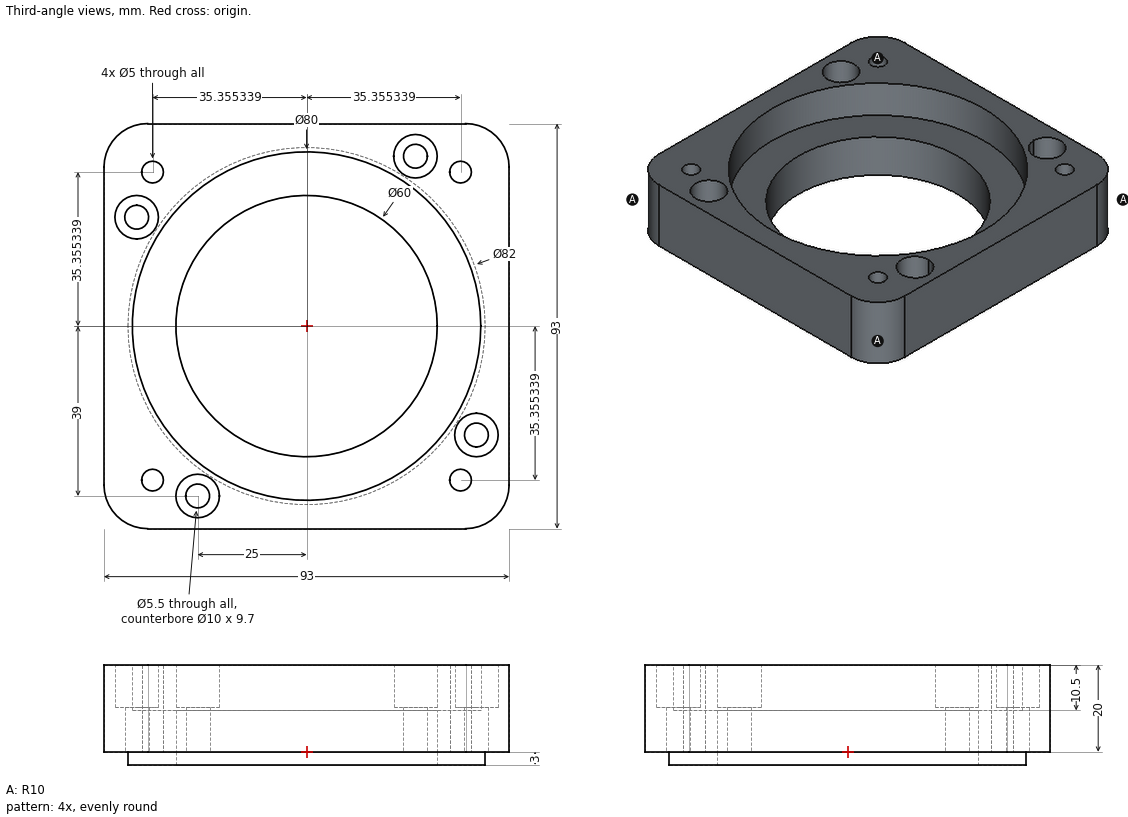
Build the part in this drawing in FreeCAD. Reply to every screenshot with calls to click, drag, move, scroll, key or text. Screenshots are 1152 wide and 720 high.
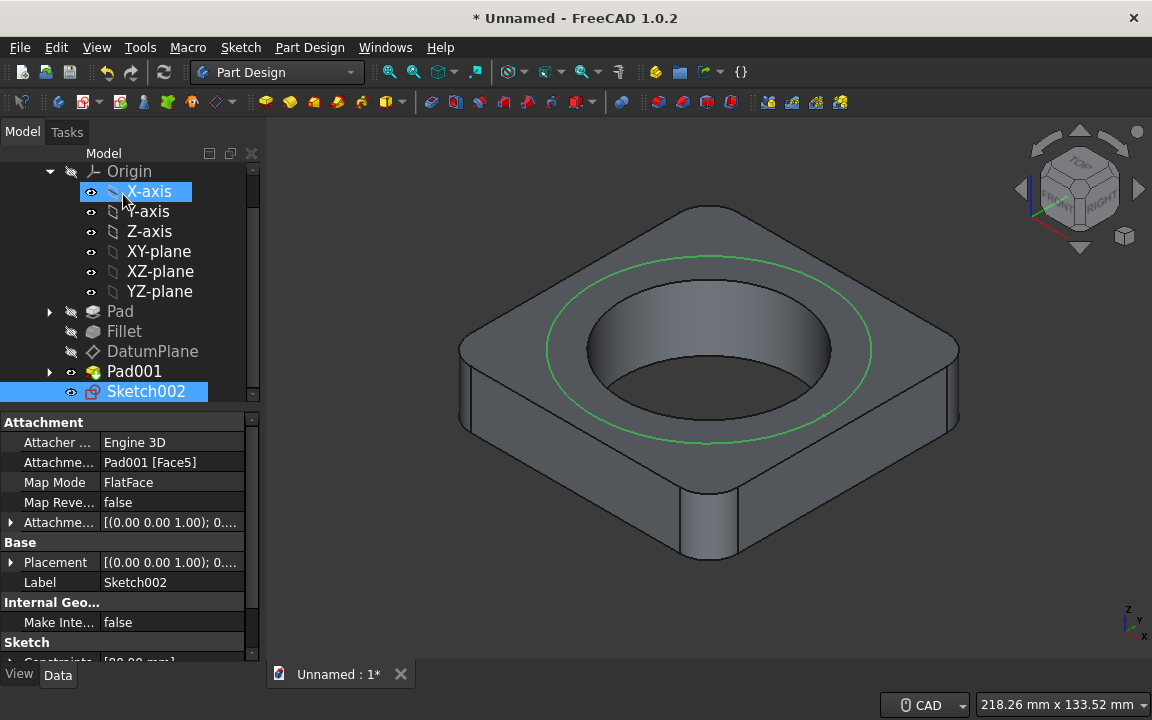
click(432, 102)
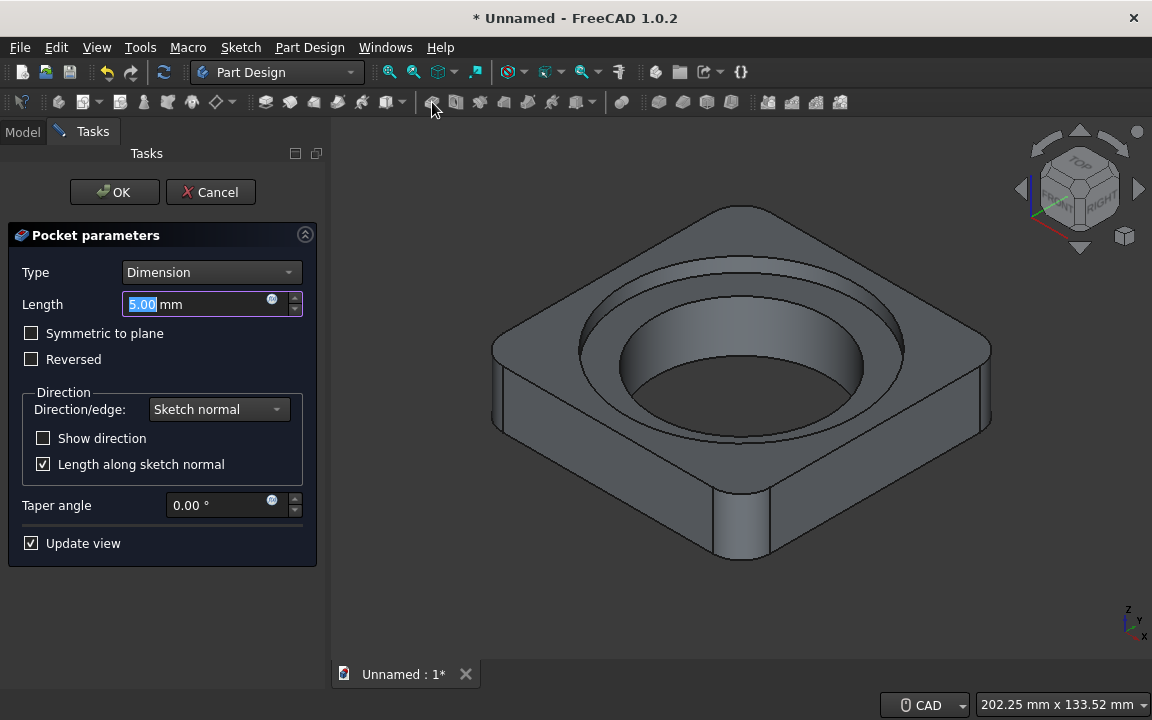
text(10.5)
key(Tab)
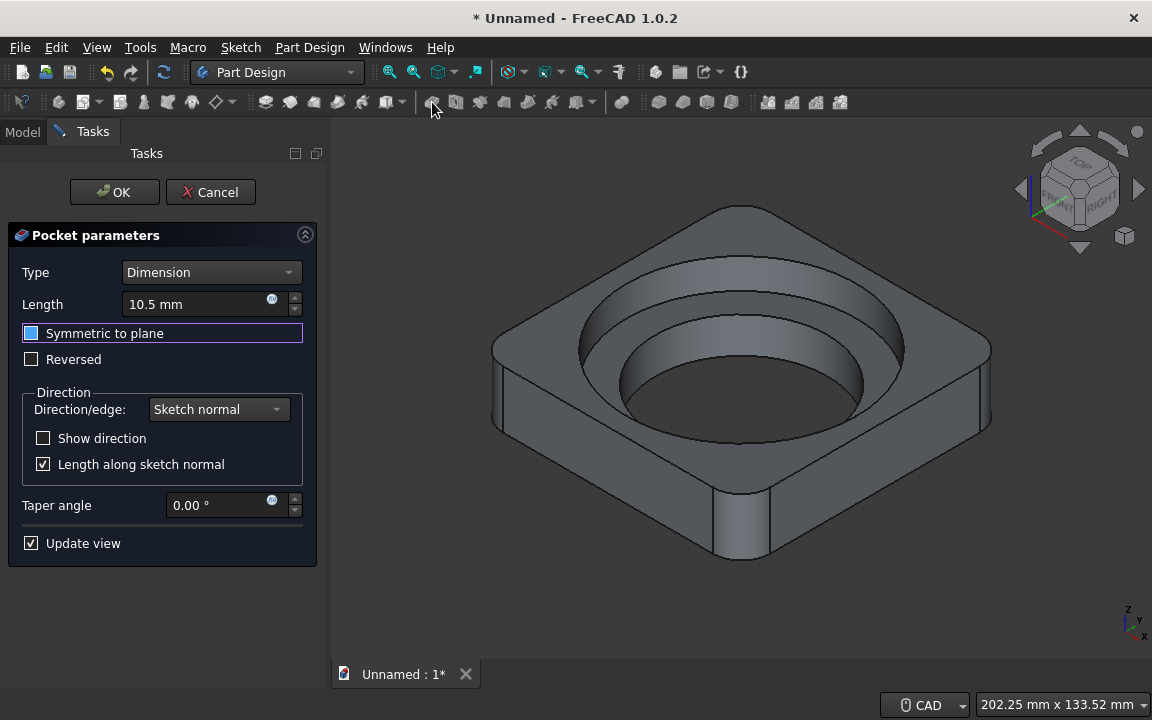
click(115, 192)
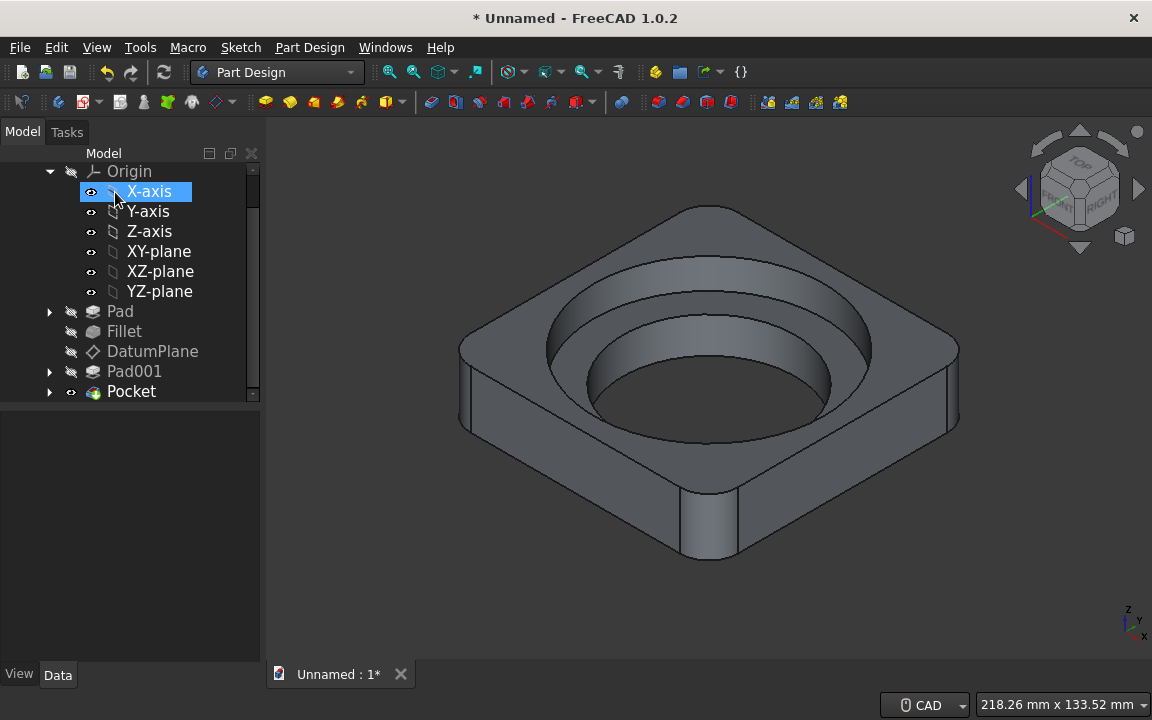
click(671, 459)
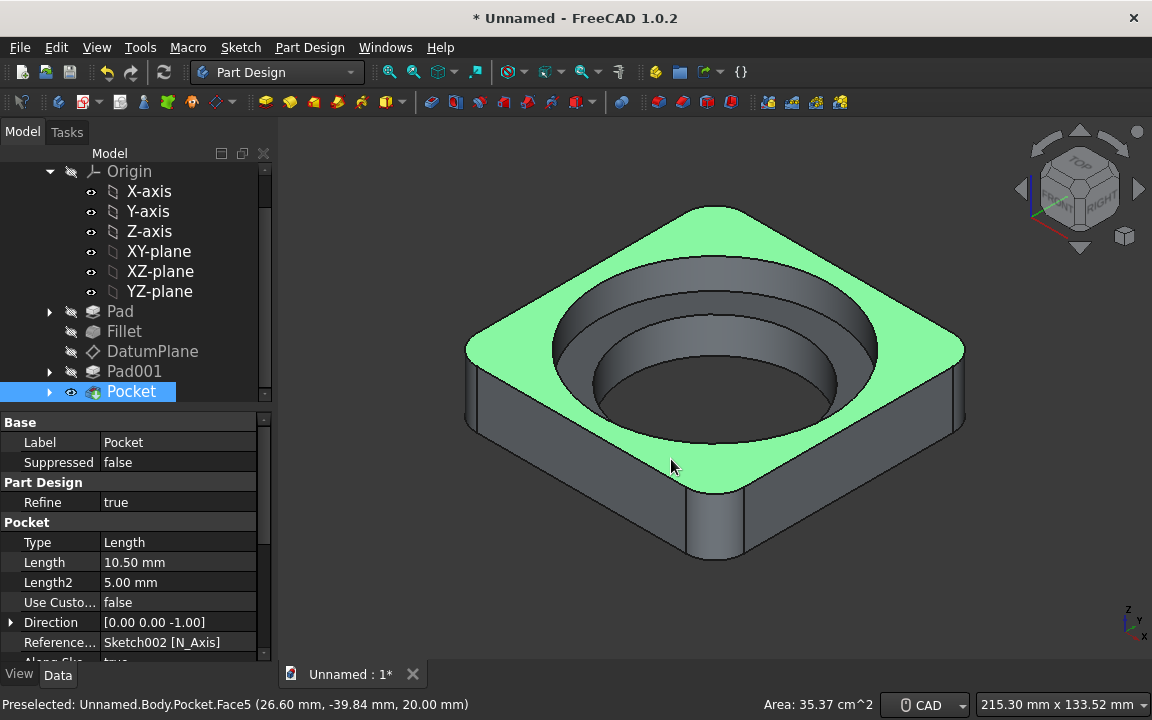
click(84, 102)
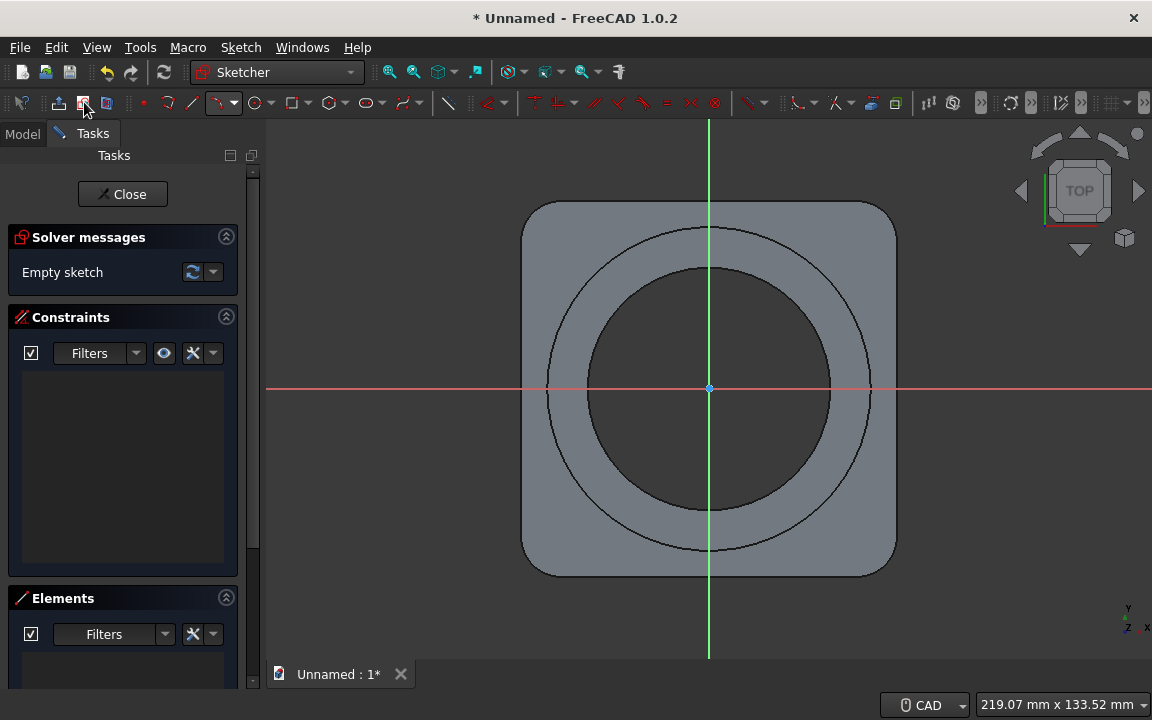
click(256, 104)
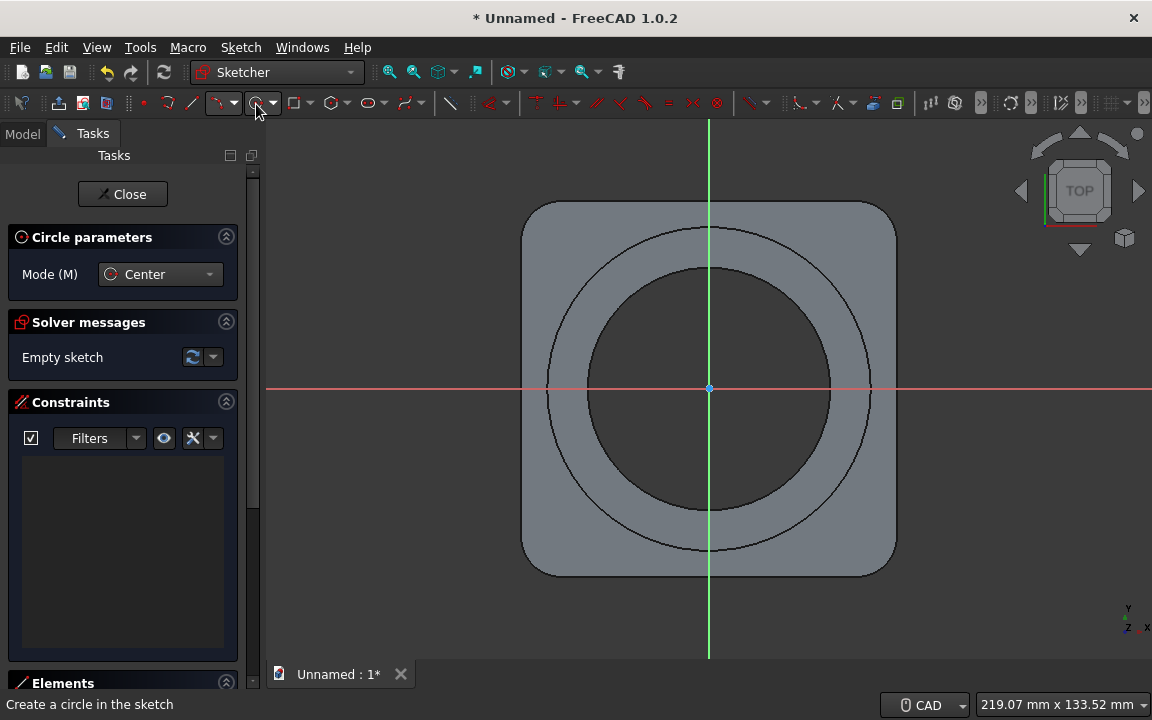
scroll(566, 246, up, 5)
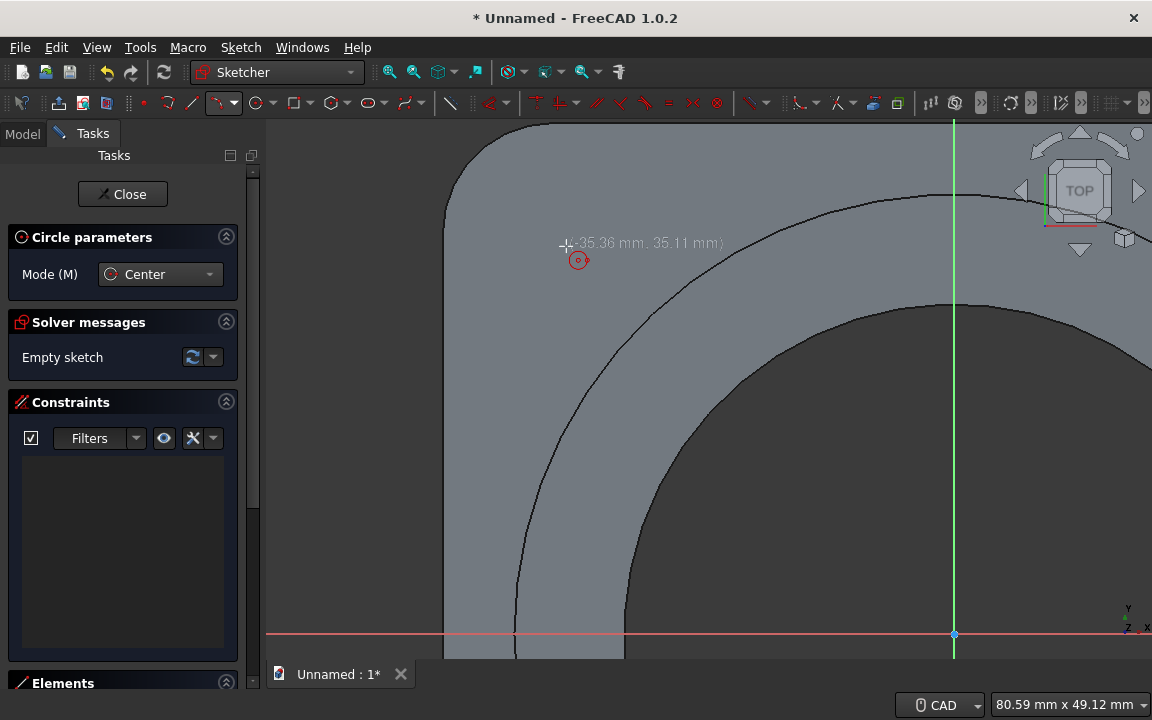
click(565, 246)
click(585, 226)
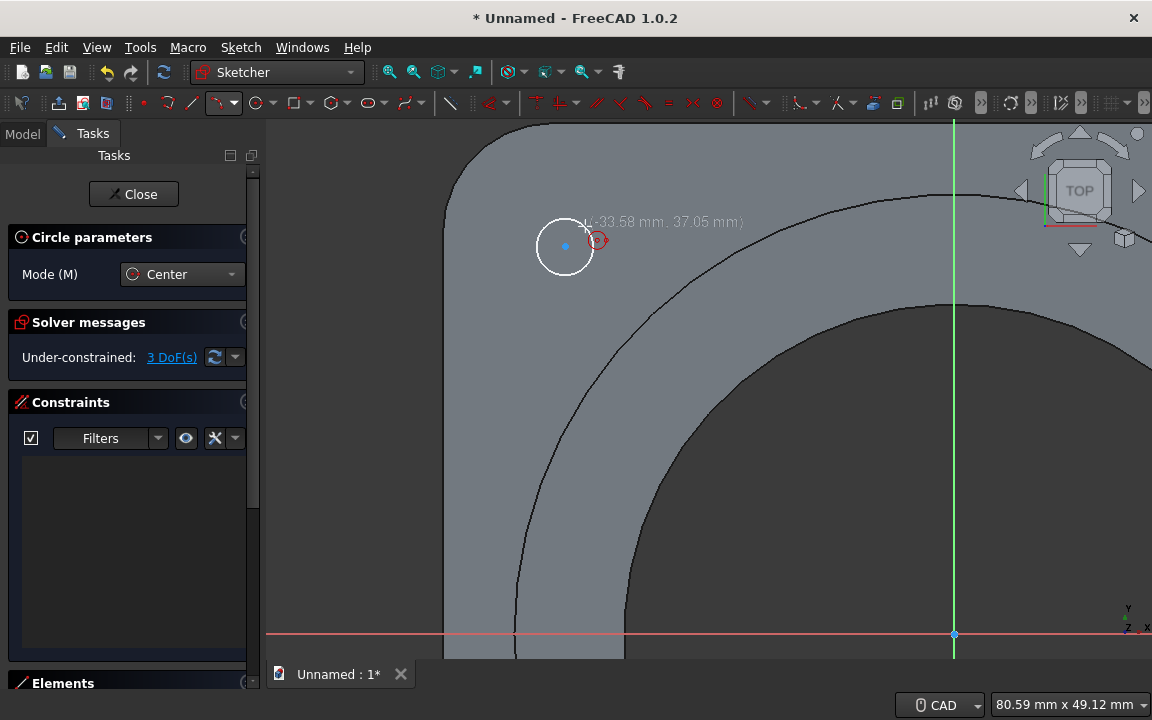
scroll(385, 189, down, 4)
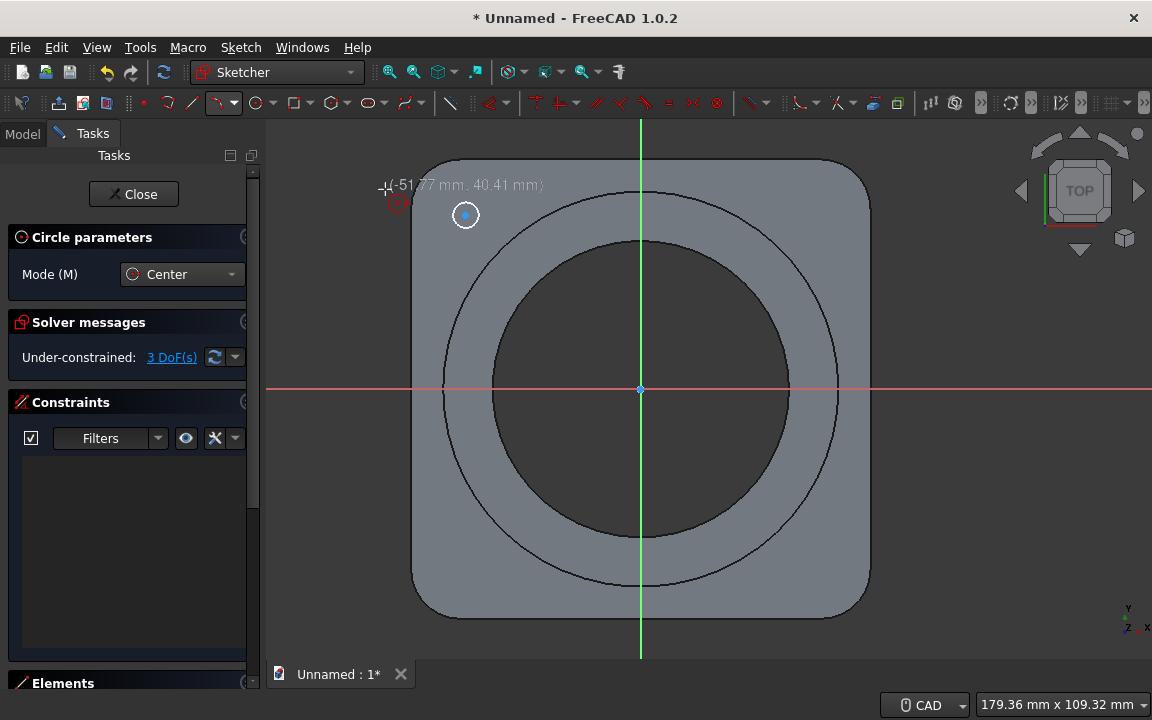
scroll(815, 215, up, 4)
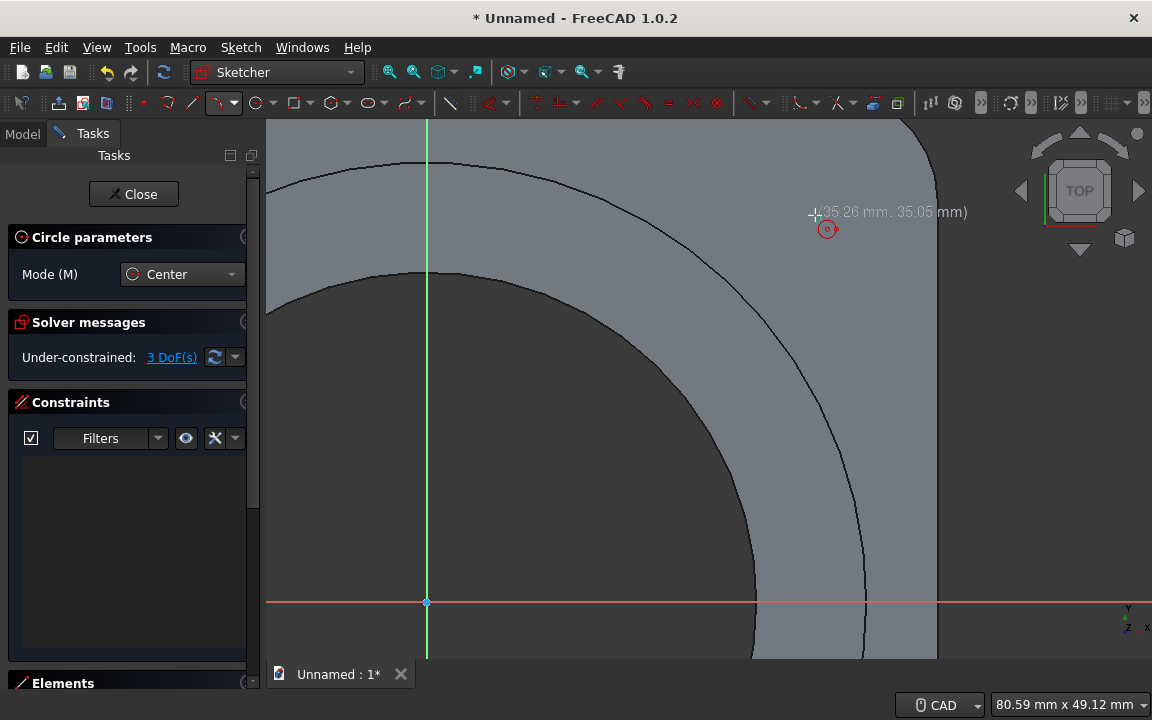
click(815, 214)
click(835, 194)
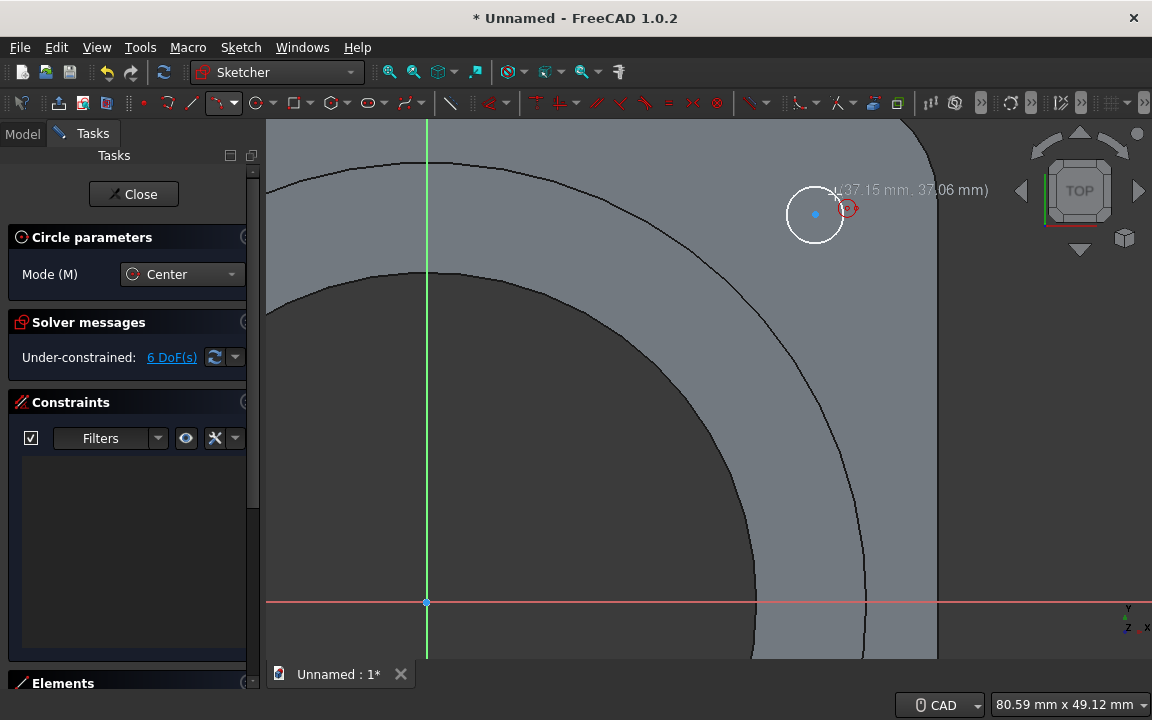
scroll(815, 215, down, 4)